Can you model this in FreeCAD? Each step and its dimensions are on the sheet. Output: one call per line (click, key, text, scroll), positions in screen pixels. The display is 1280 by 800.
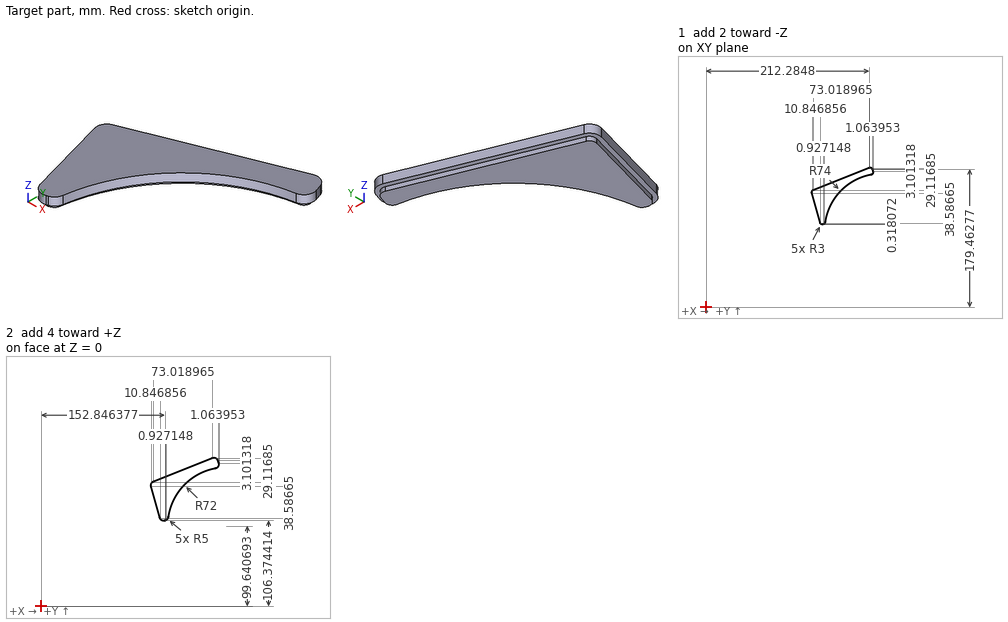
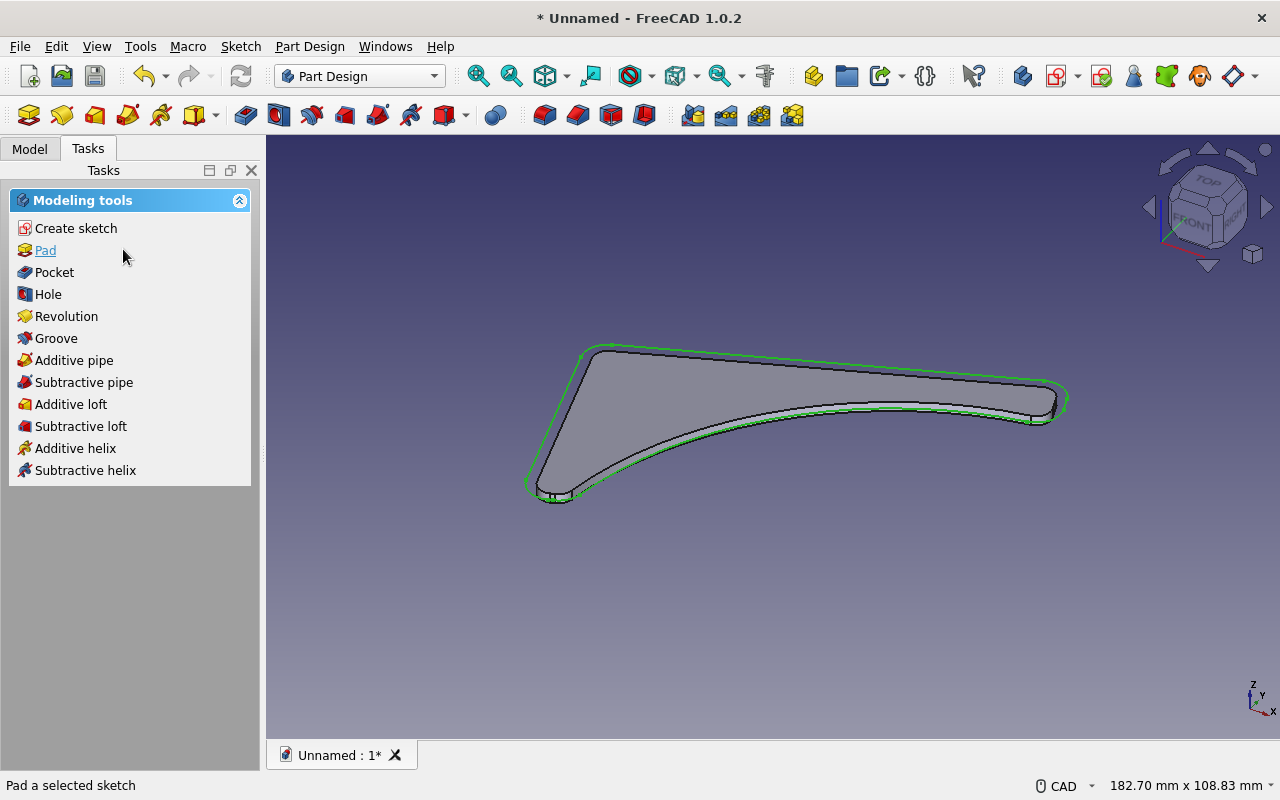
click(29, 116)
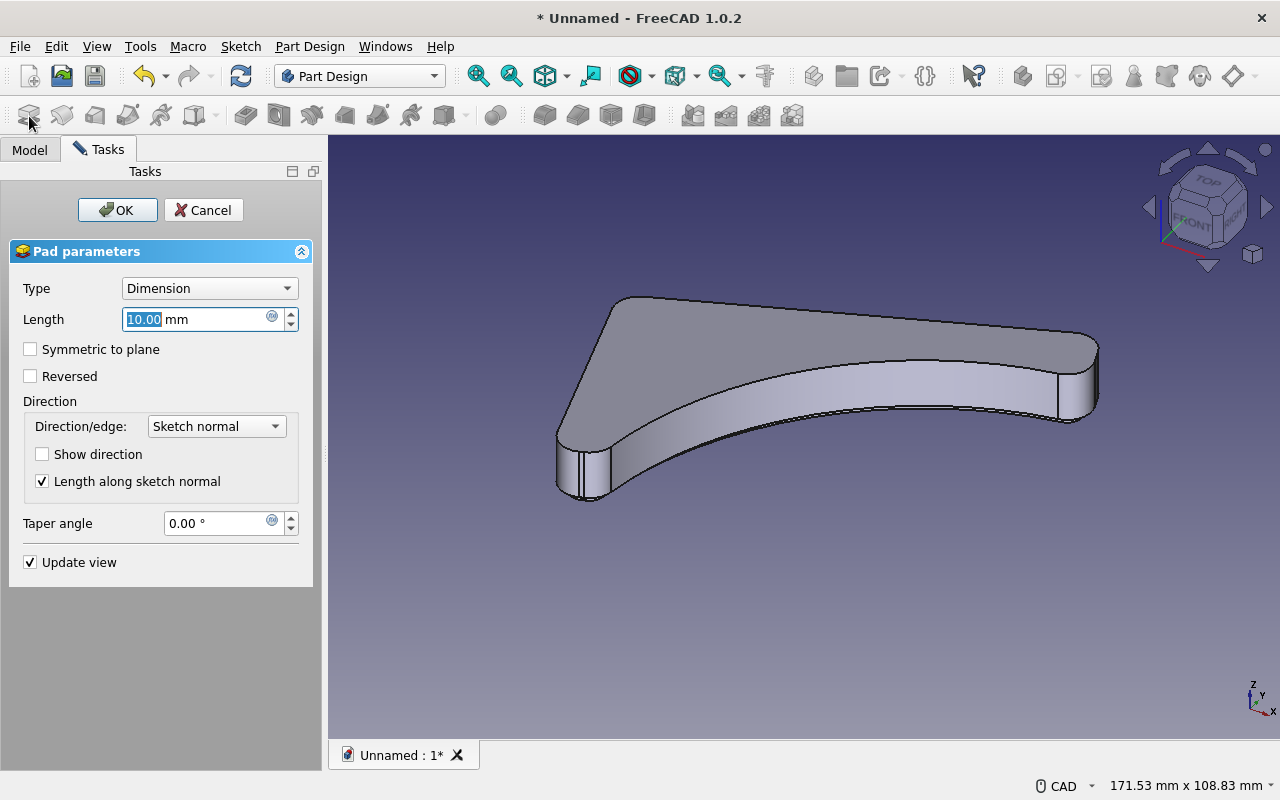
text(4)
key(Tab)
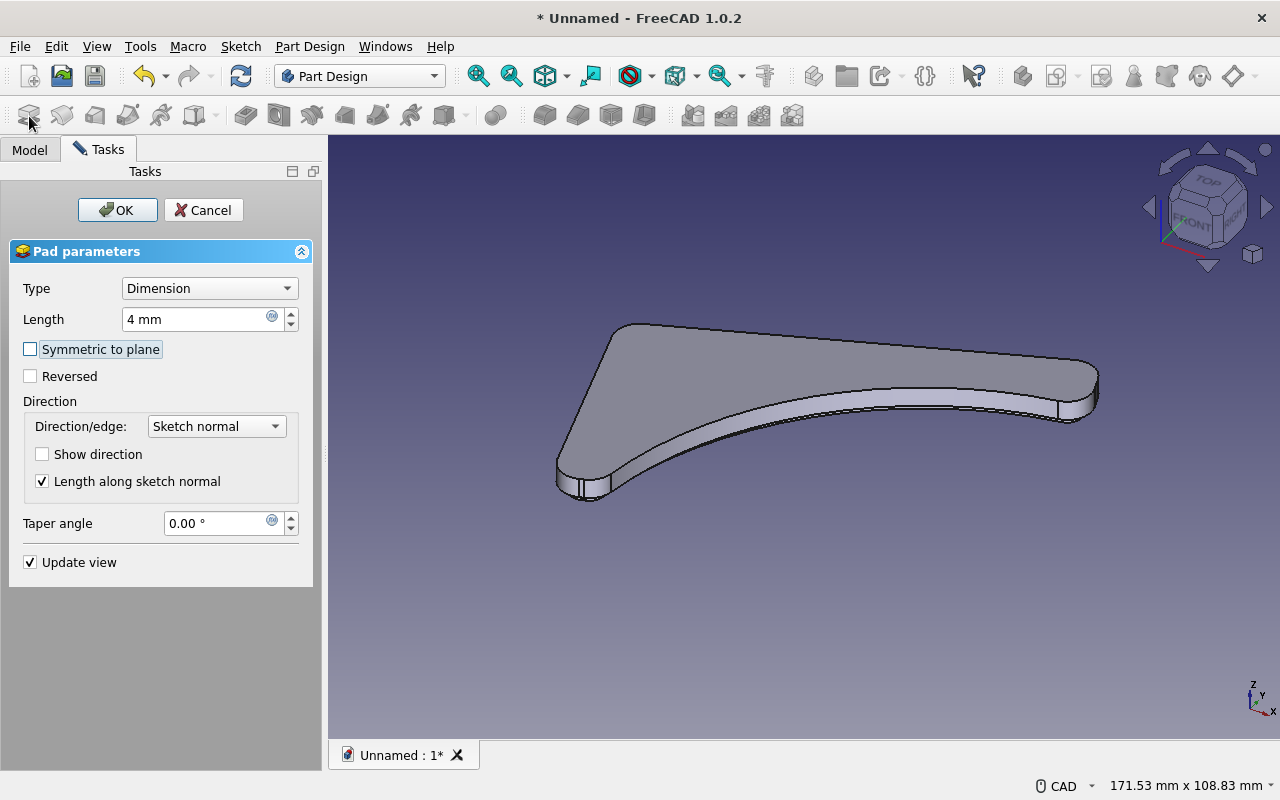
click(118, 210)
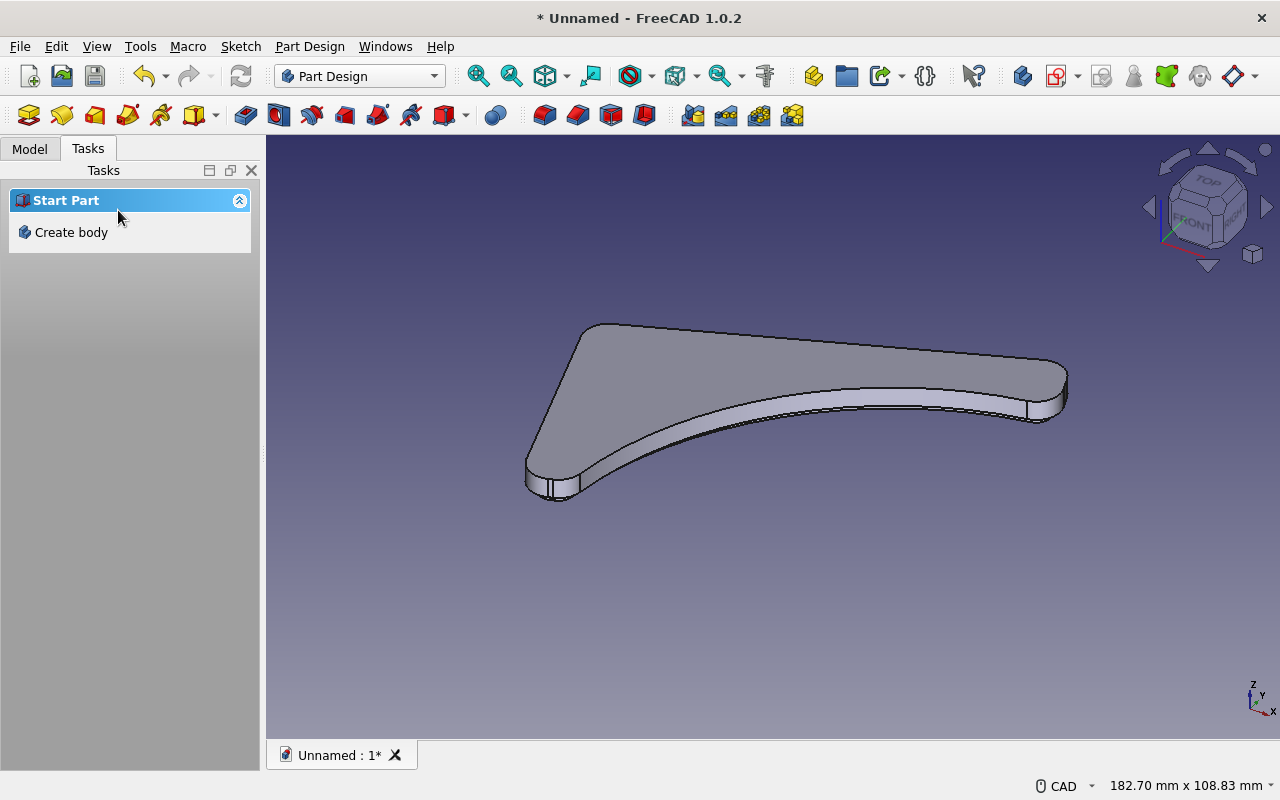
key(0)